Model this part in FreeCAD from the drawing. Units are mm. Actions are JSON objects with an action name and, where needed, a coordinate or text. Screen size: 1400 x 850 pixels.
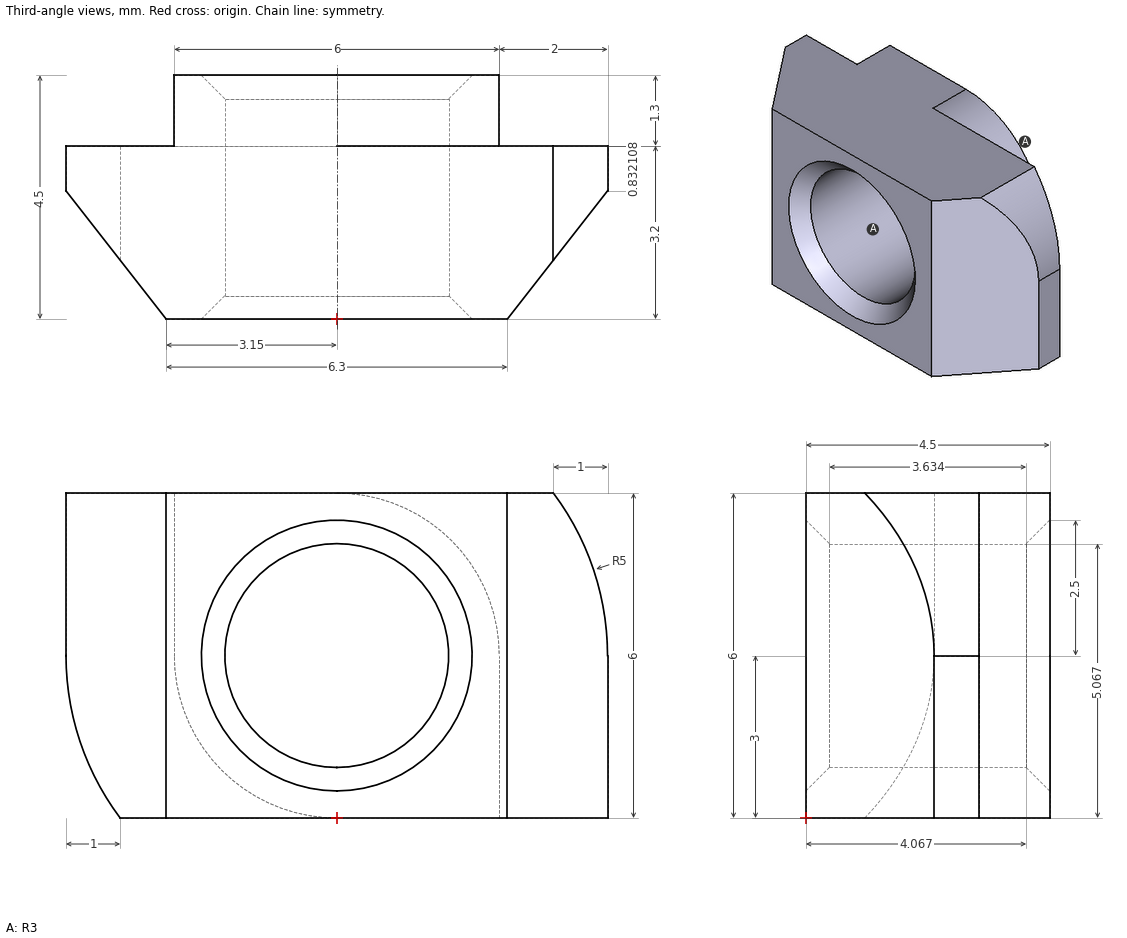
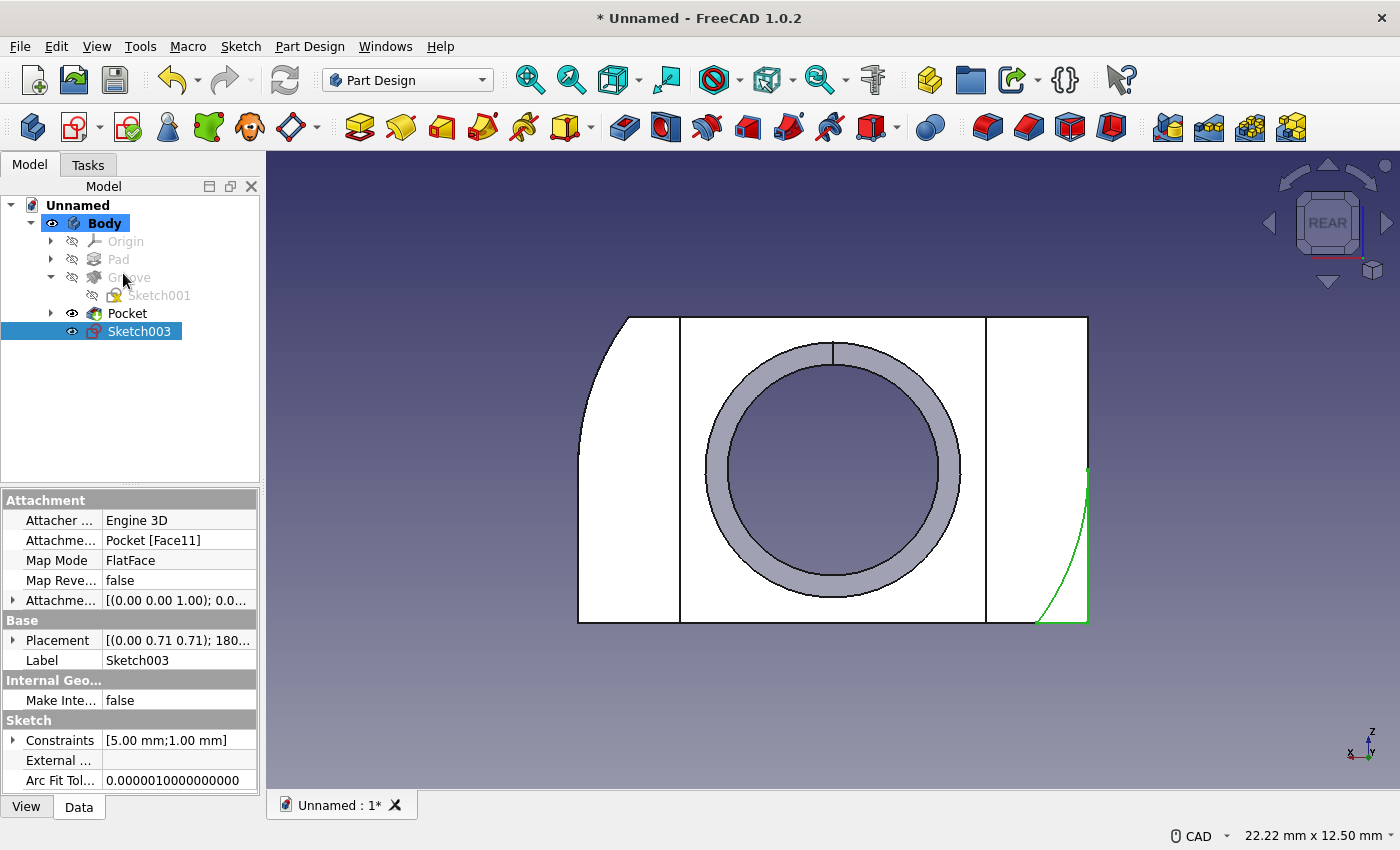
{"action": "left_click", "coordinate": [625, 128]}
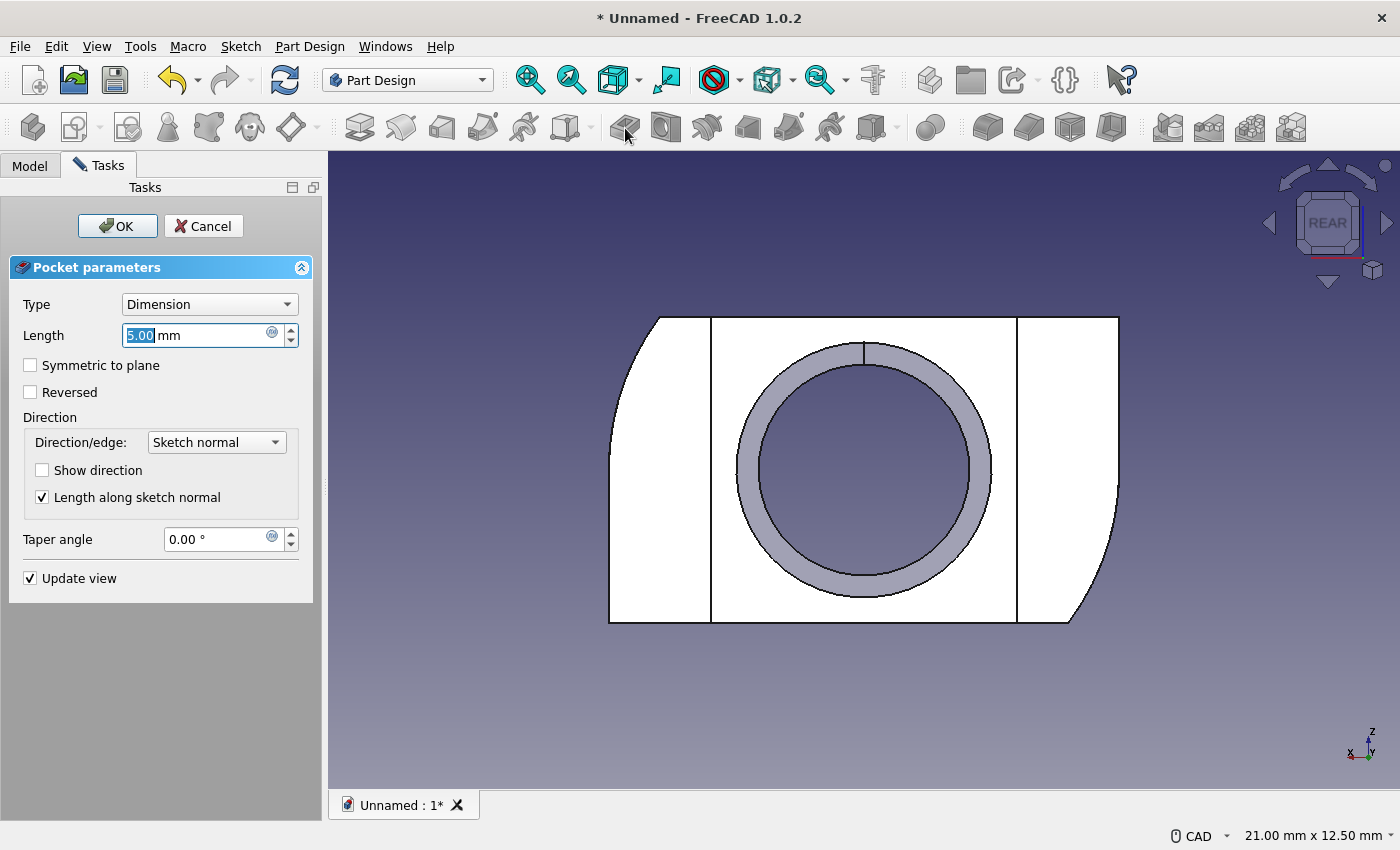
{"action": "type", "text": "4.5"}
{"action": "key", "text": "Tab"}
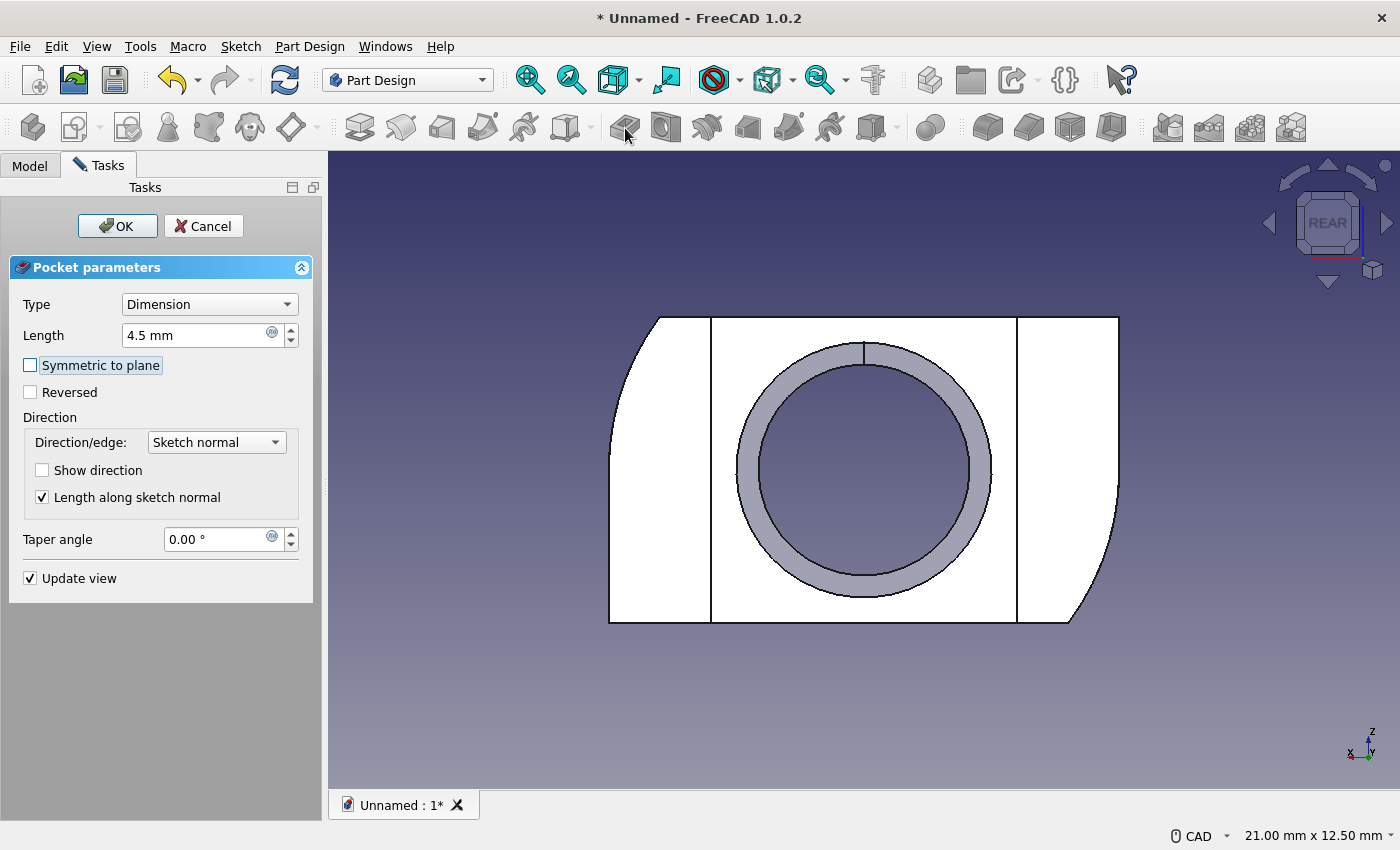
{"action": "left_click", "coordinate": [118, 226]}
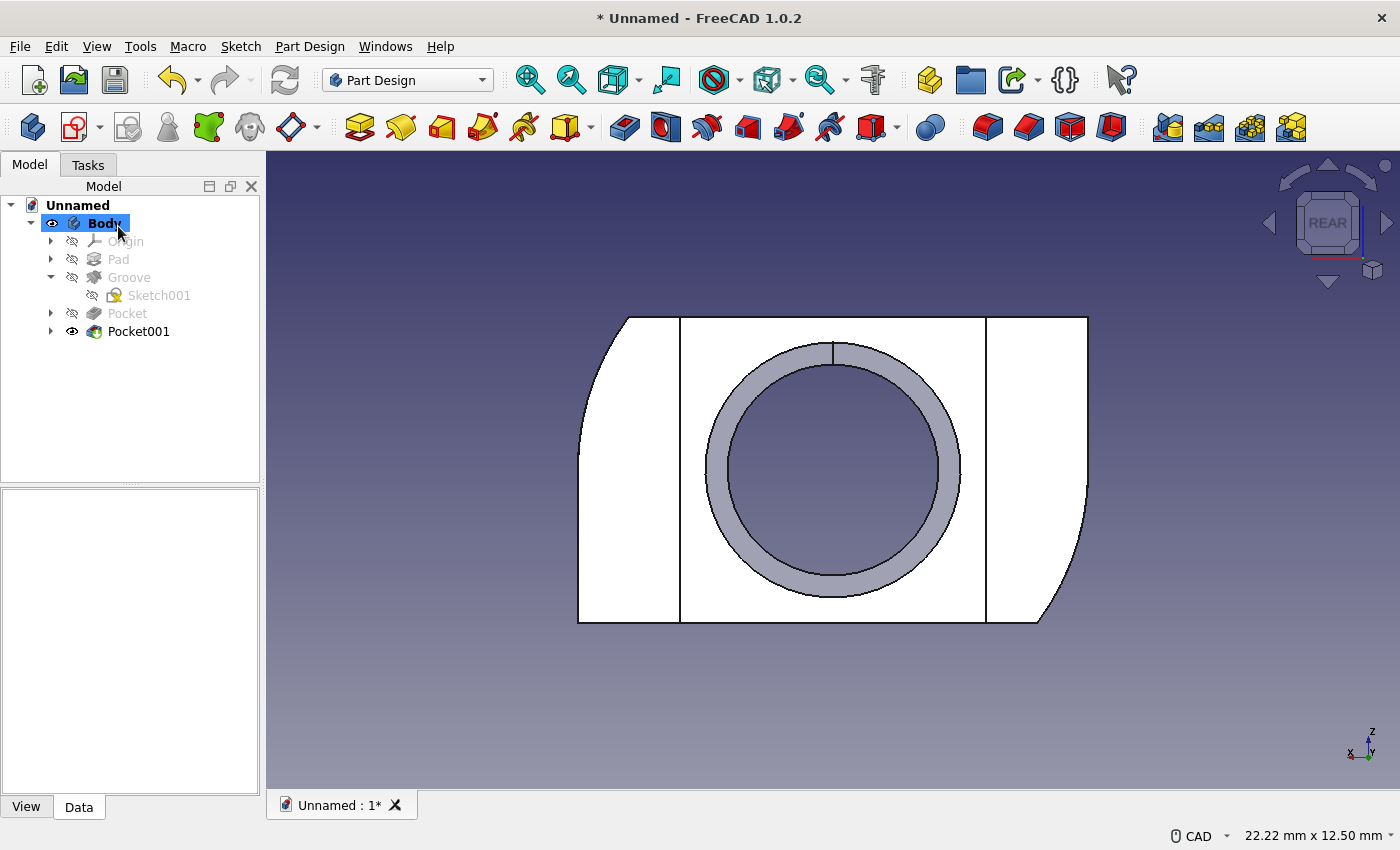
{"action": "key", "text": "0"}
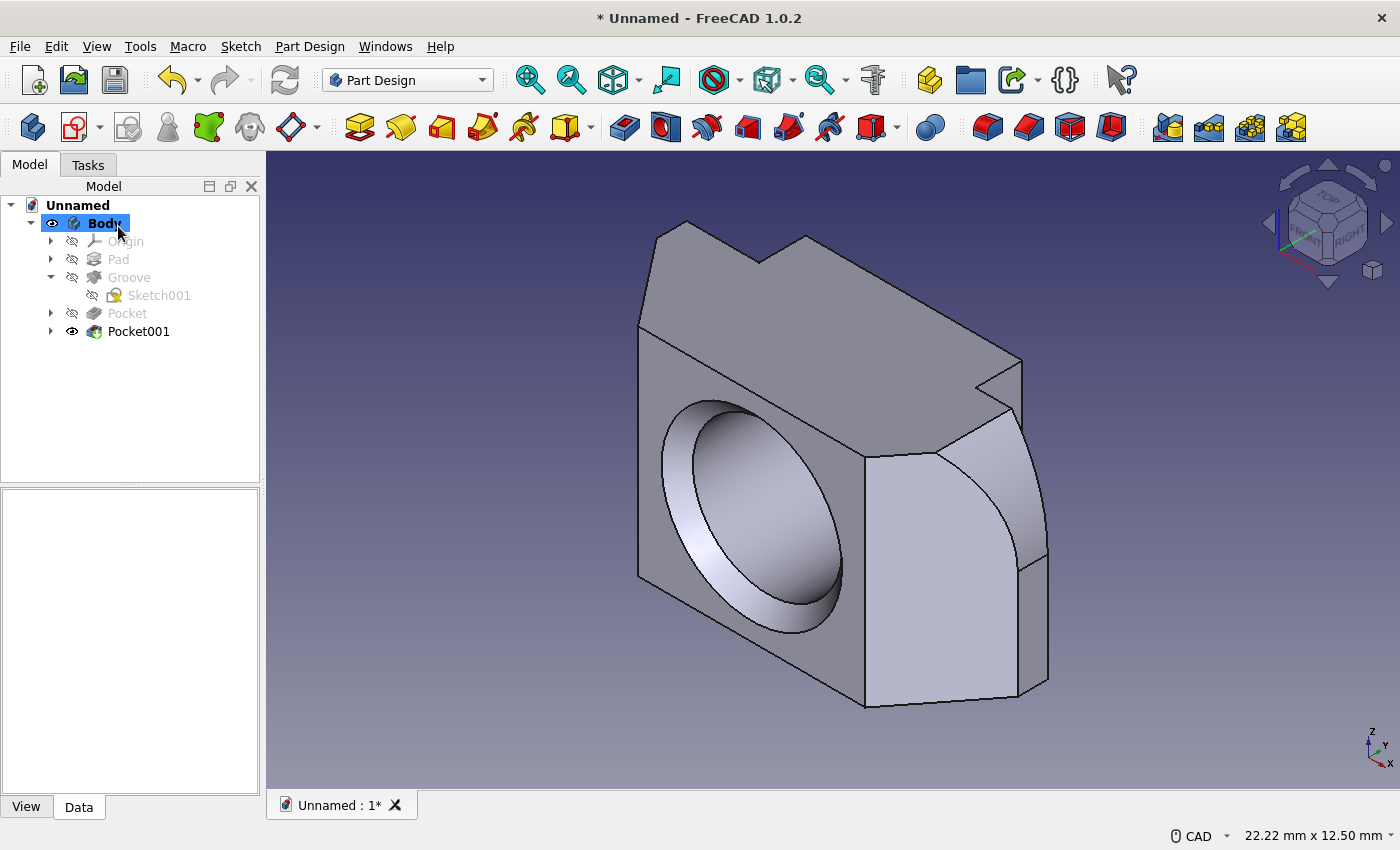
{"action": "left_click", "coordinate": [999, 373]}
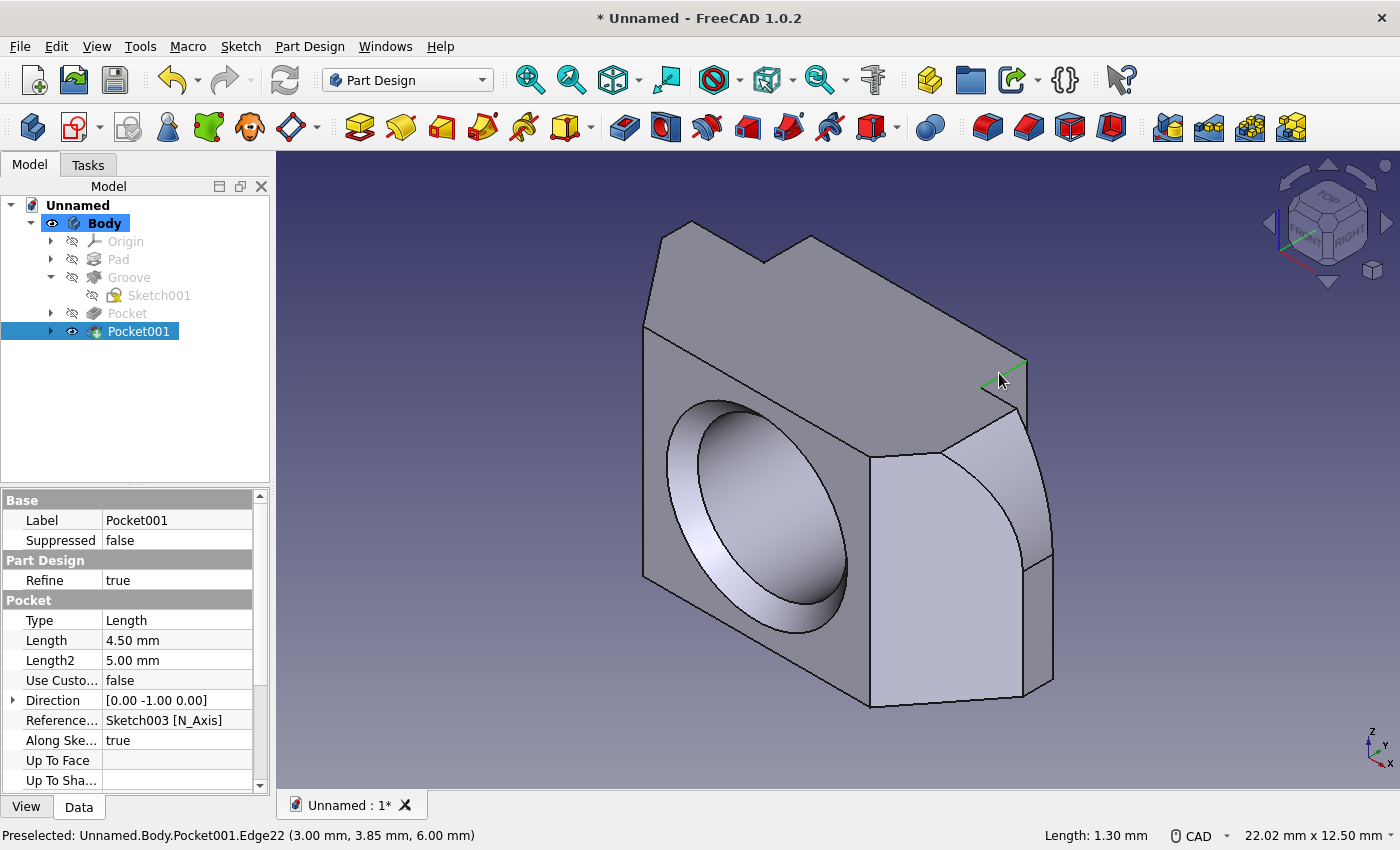
{"action": "key", "text": "2"}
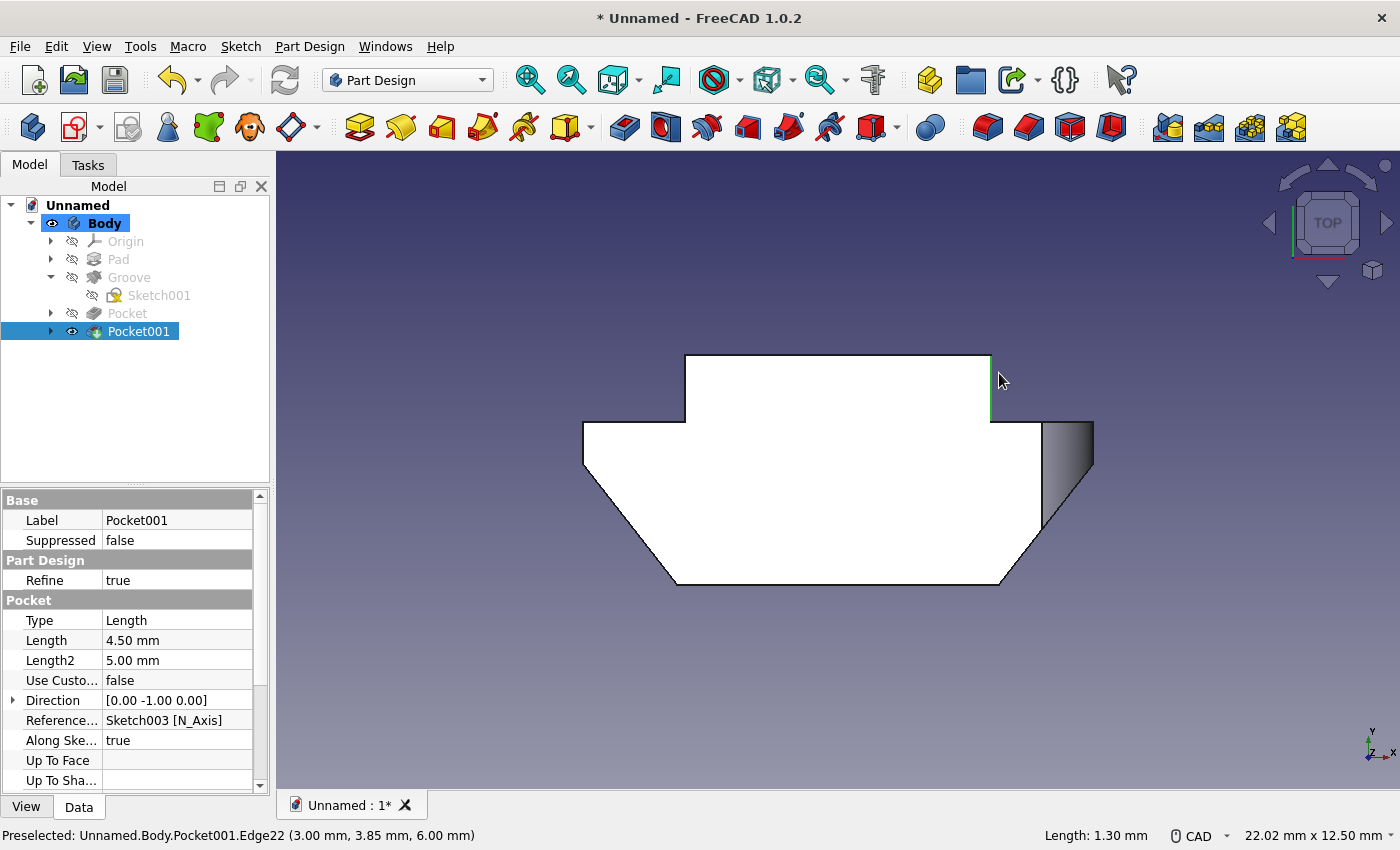
{"action": "key", "text": "1"}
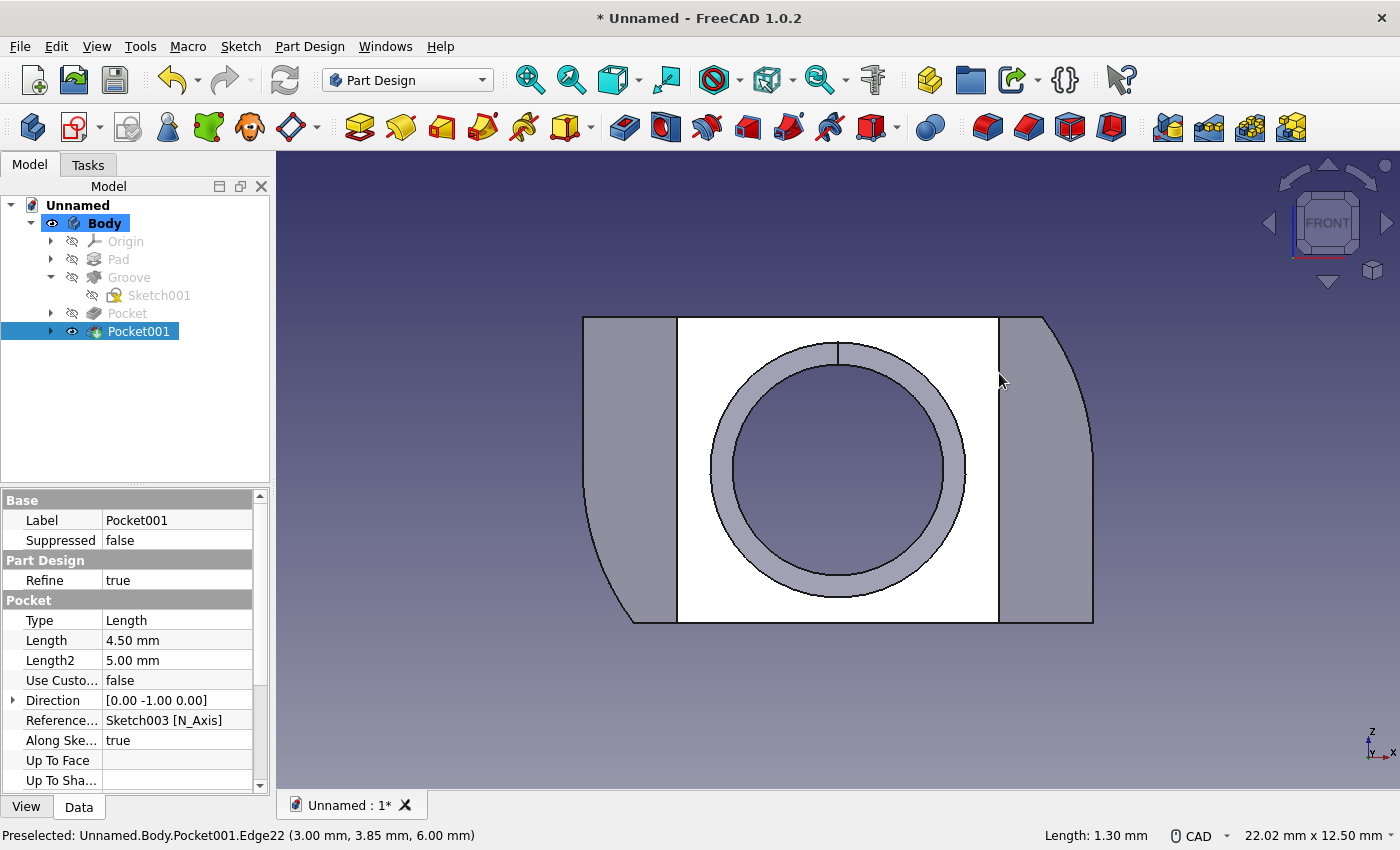
{"action": "key", "text": "3"}